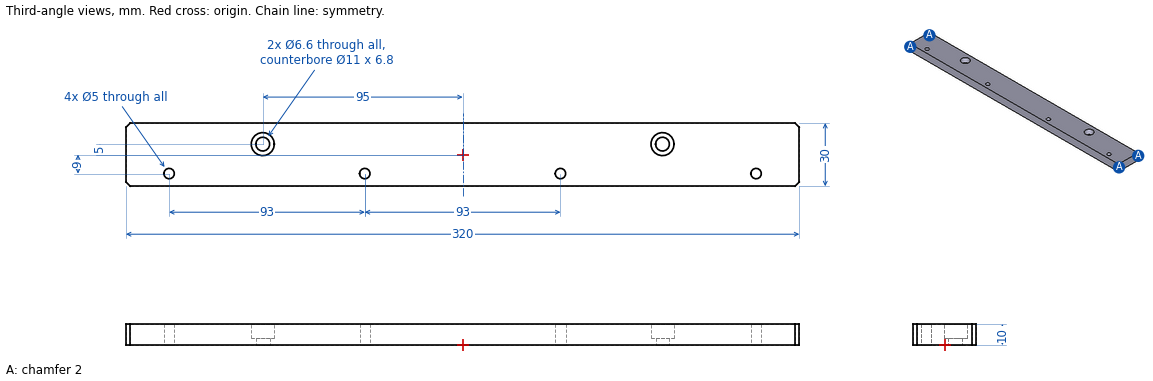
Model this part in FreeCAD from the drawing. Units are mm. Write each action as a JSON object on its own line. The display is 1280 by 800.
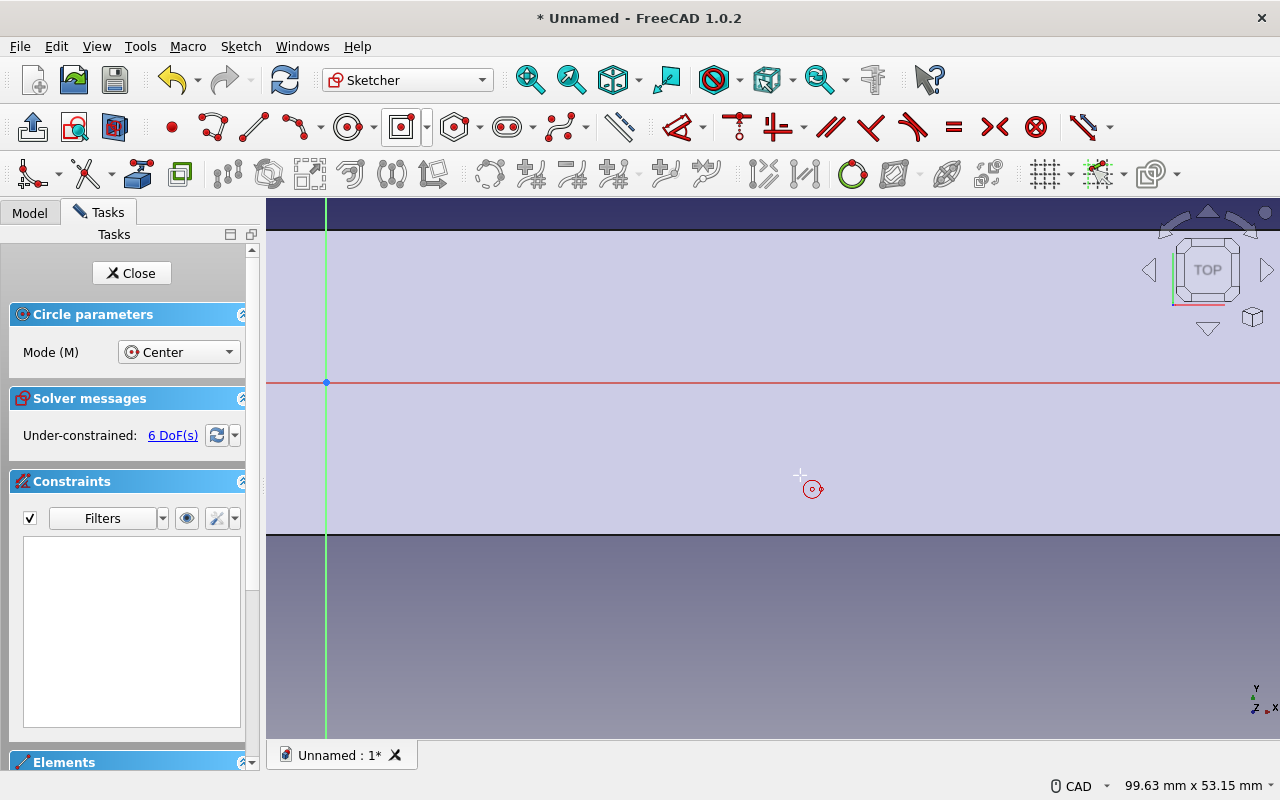
{"action": "scroll", "coordinate": [800, 475], "scroll_direction": "down", "scroll_amount": 8}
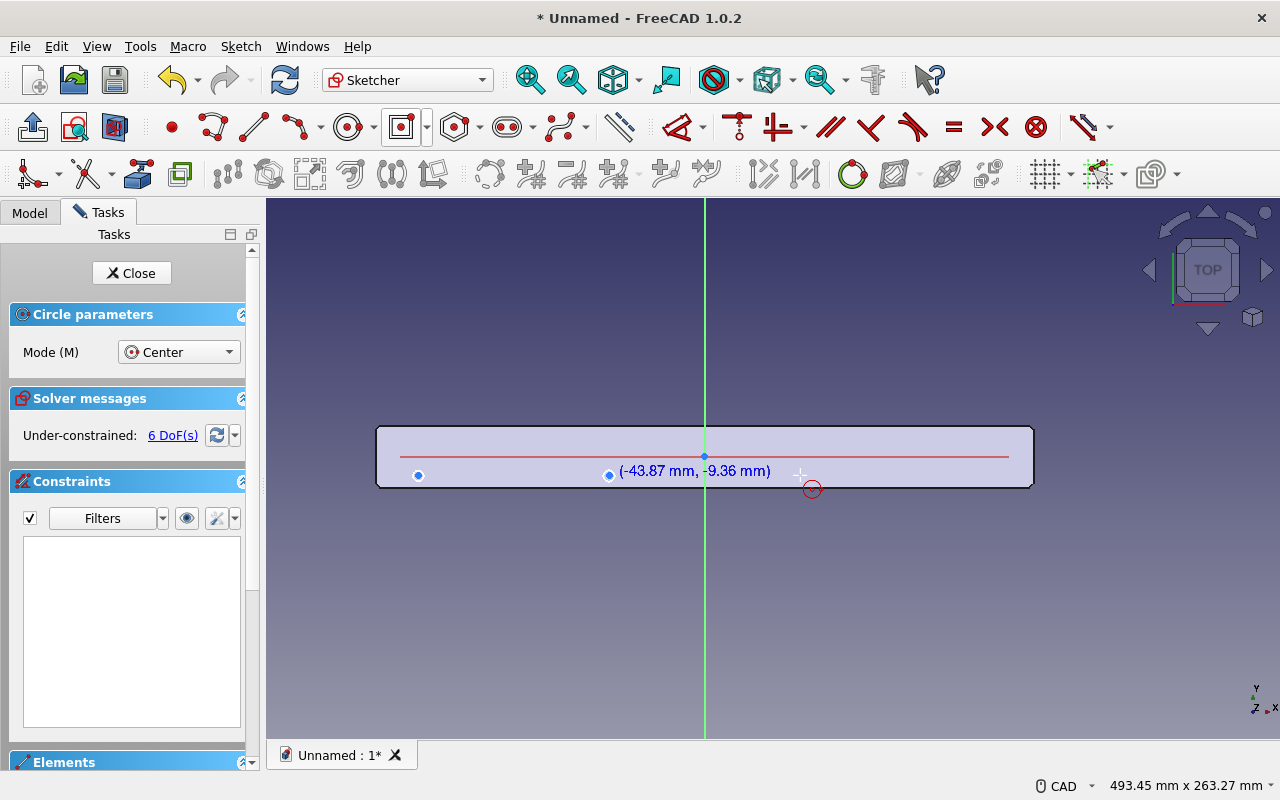
{"action": "left_click", "coordinate": [800, 475]}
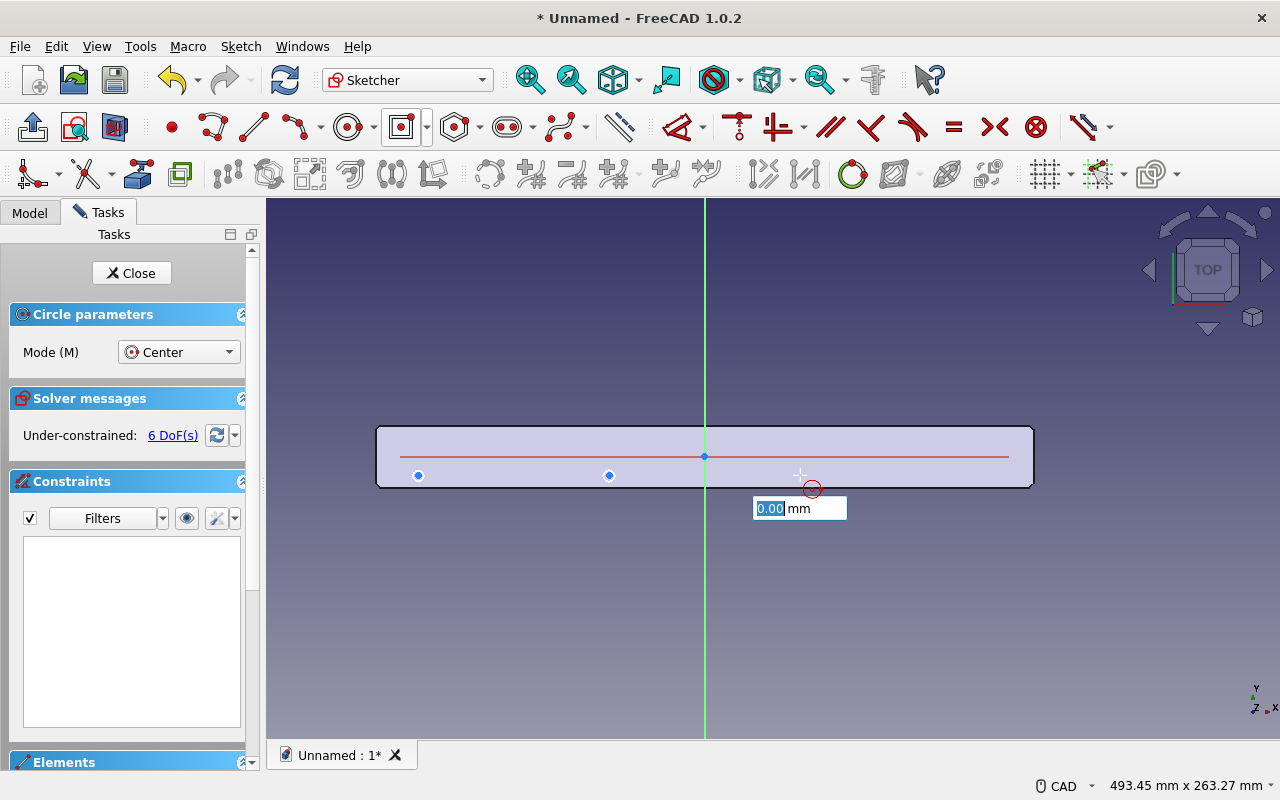
{"action": "scroll", "coordinate": [804, 472], "scroll_direction": "up", "scroll_amount": 6}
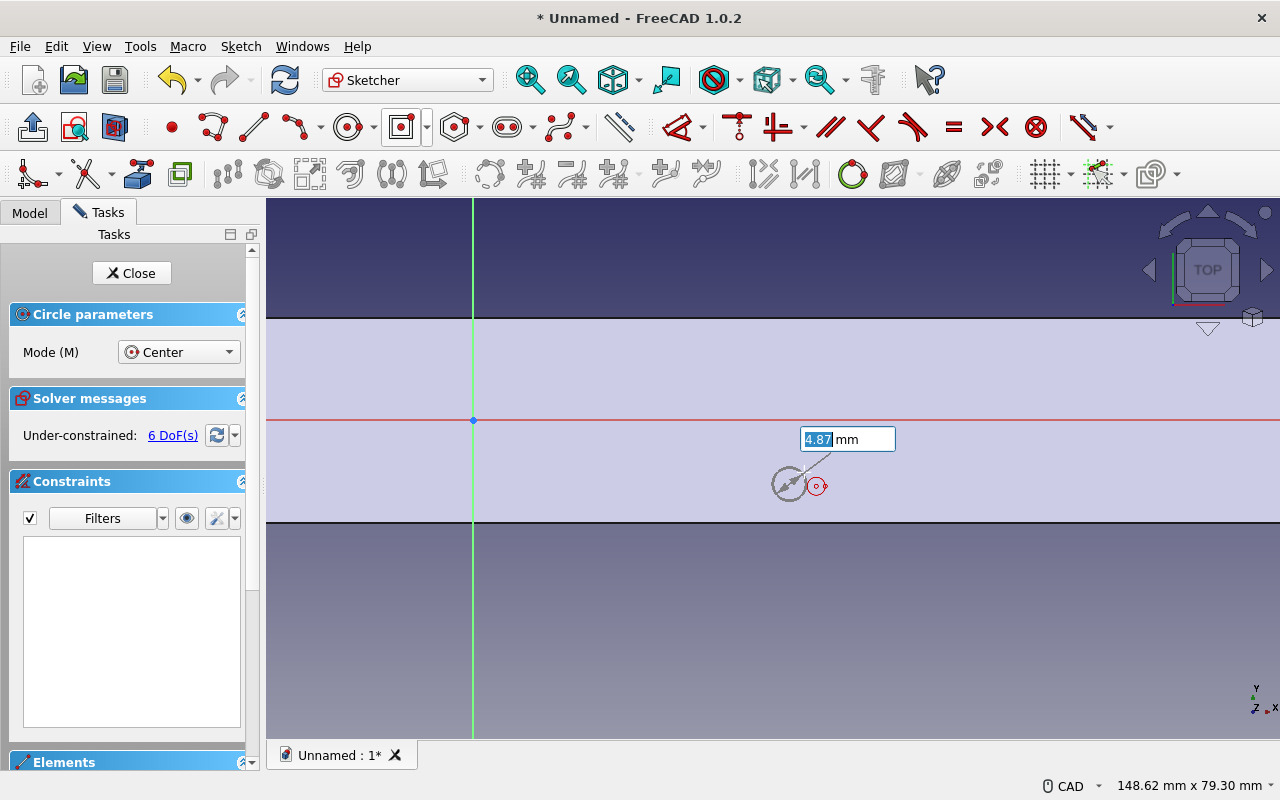
{"action": "left_click", "coordinate": [802, 470]}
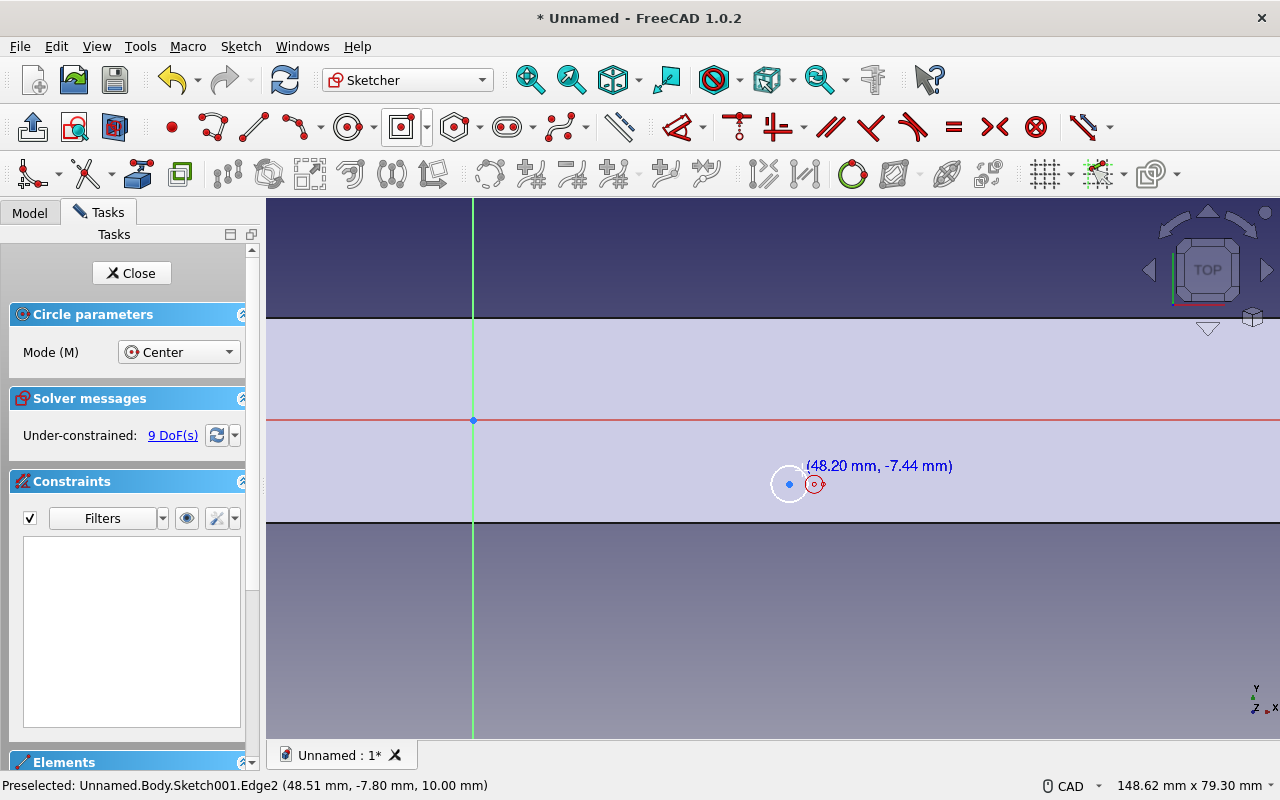
{"action": "scroll", "coordinate": [804, 472], "scroll_direction": "down", "scroll_amount": 6}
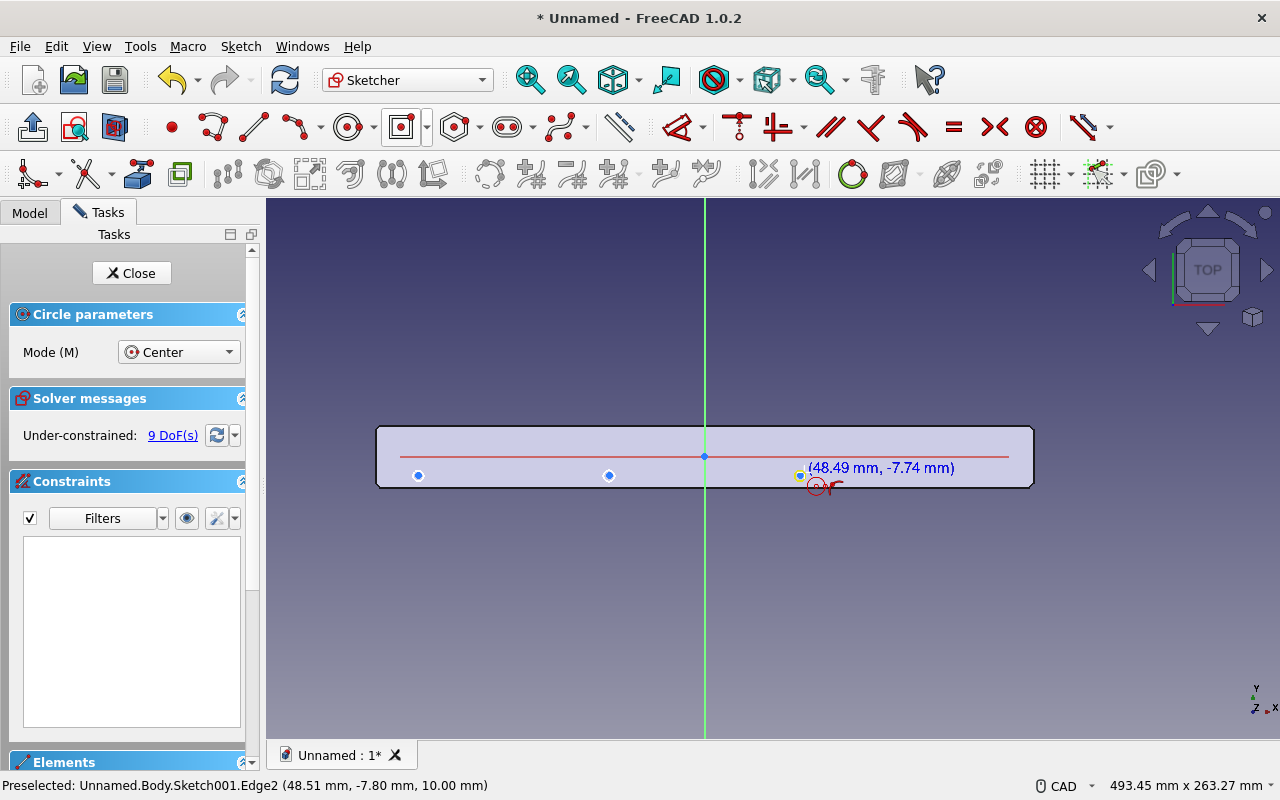
{"action": "scroll", "coordinate": [991, 475], "scroll_direction": "up", "scroll_amount": 8}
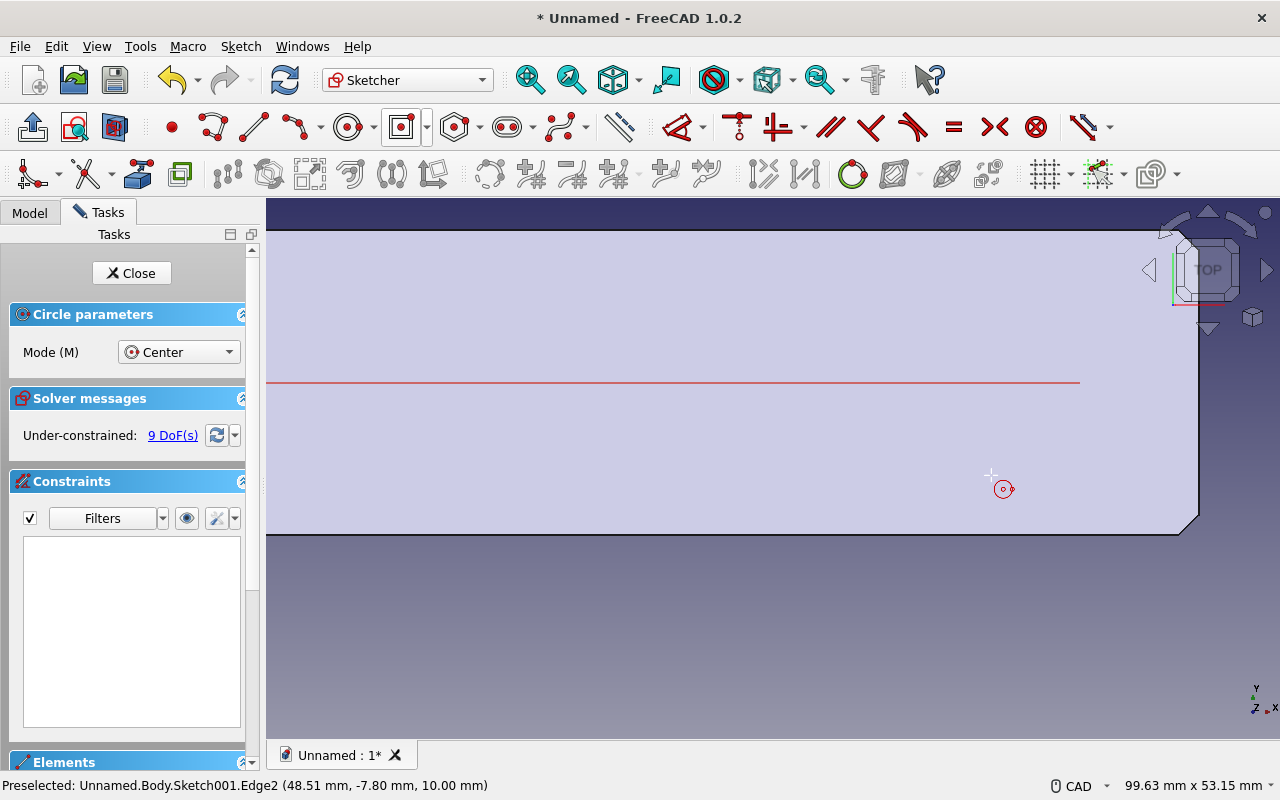
{"action": "scroll", "coordinate": [991, 475], "scroll_direction": "down", "scroll_amount": 8}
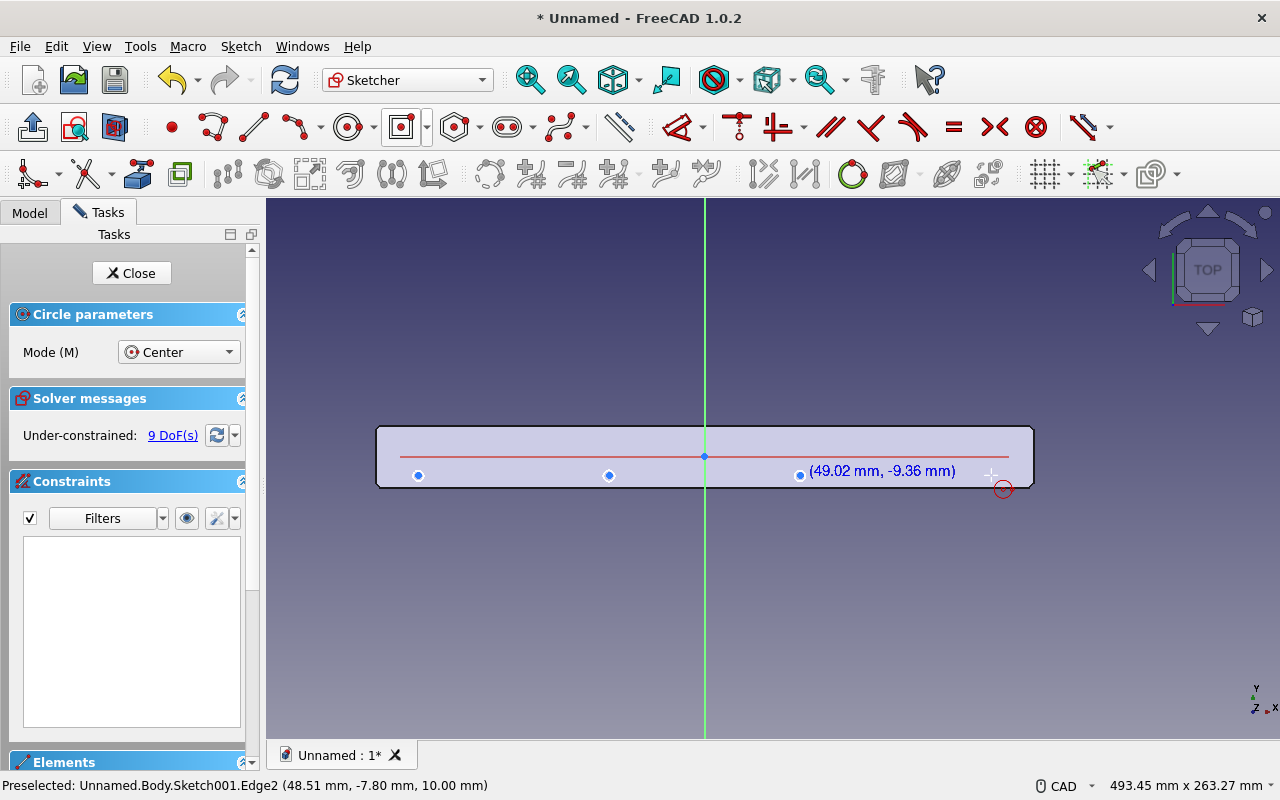
{"action": "left_click", "coordinate": [991, 475]}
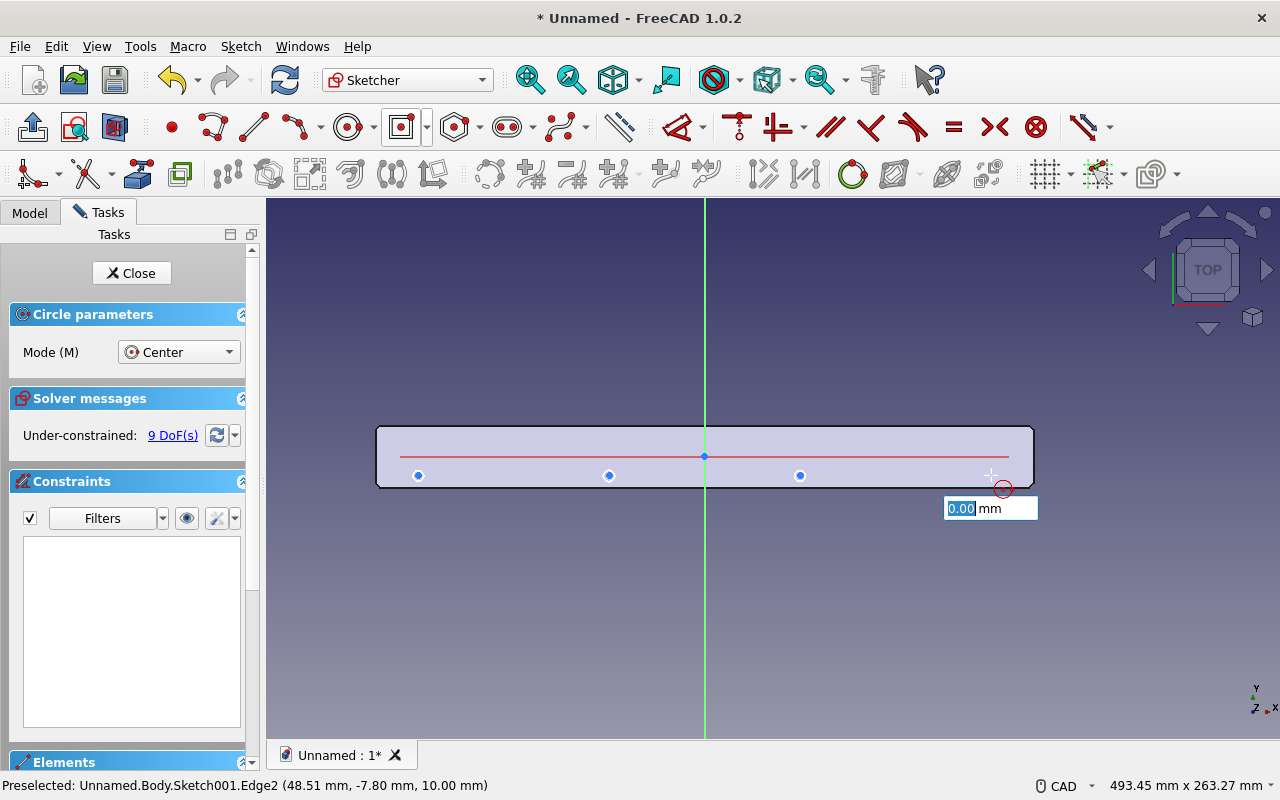
{"action": "scroll", "coordinate": [995, 472], "scroll_direction": "up", "scroll_amount": 6}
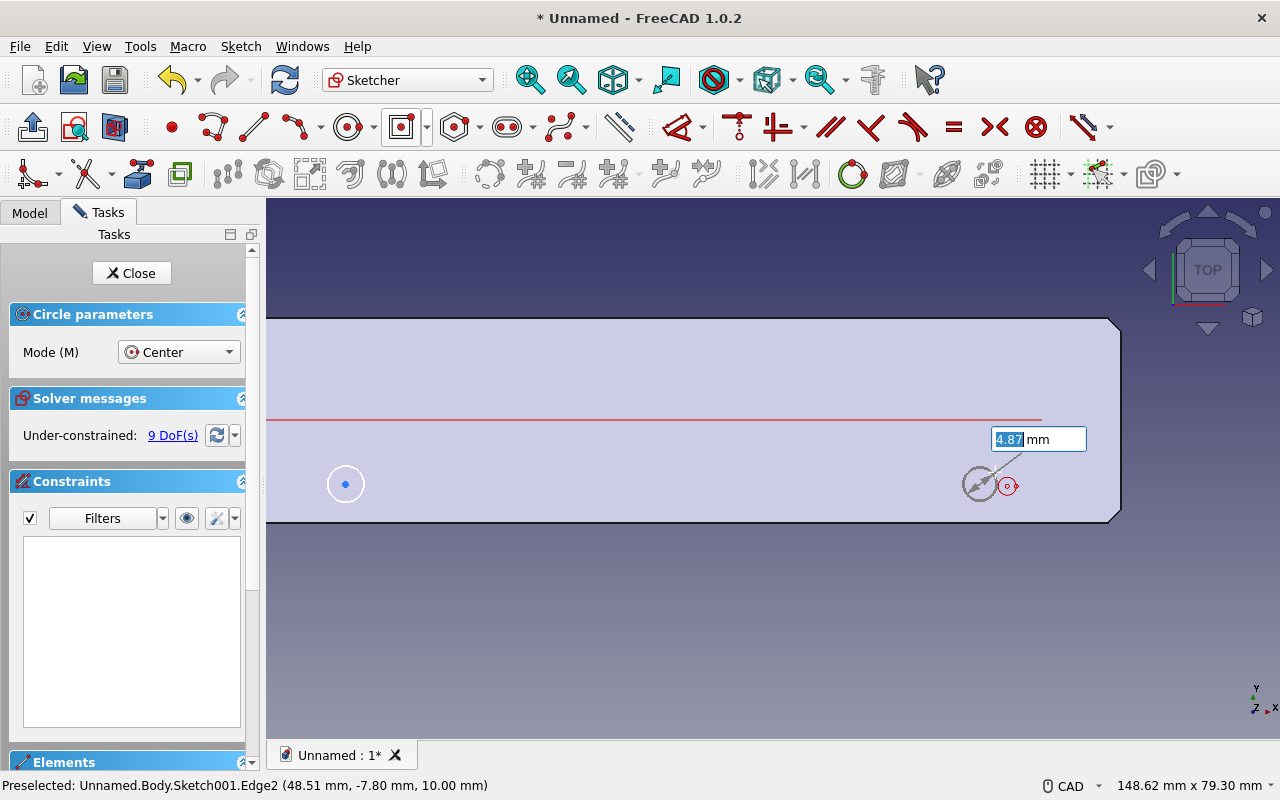
{"action": "left_click", "coordinate": [993, 470]}
{"action": "key", "text": "Escape"}